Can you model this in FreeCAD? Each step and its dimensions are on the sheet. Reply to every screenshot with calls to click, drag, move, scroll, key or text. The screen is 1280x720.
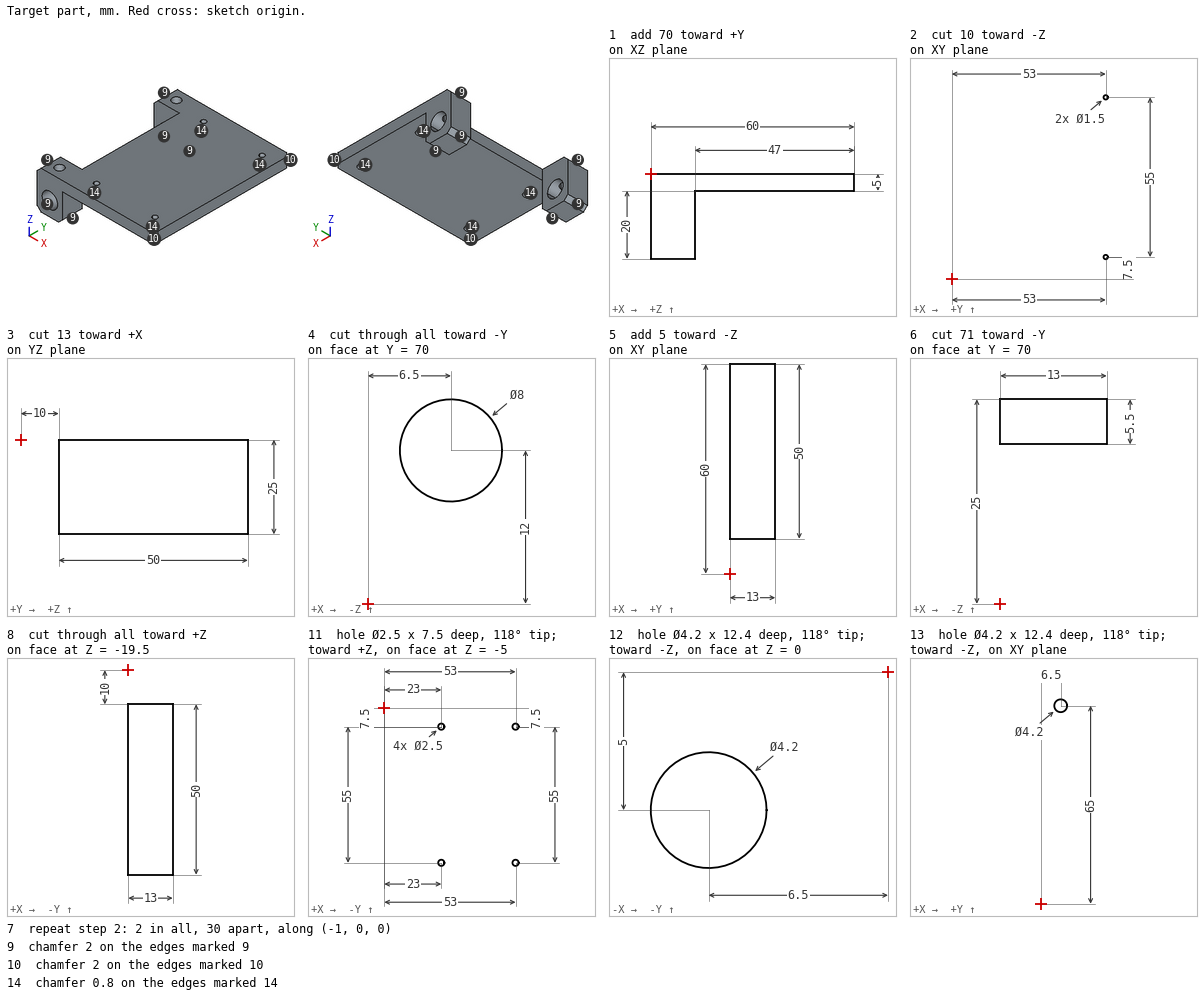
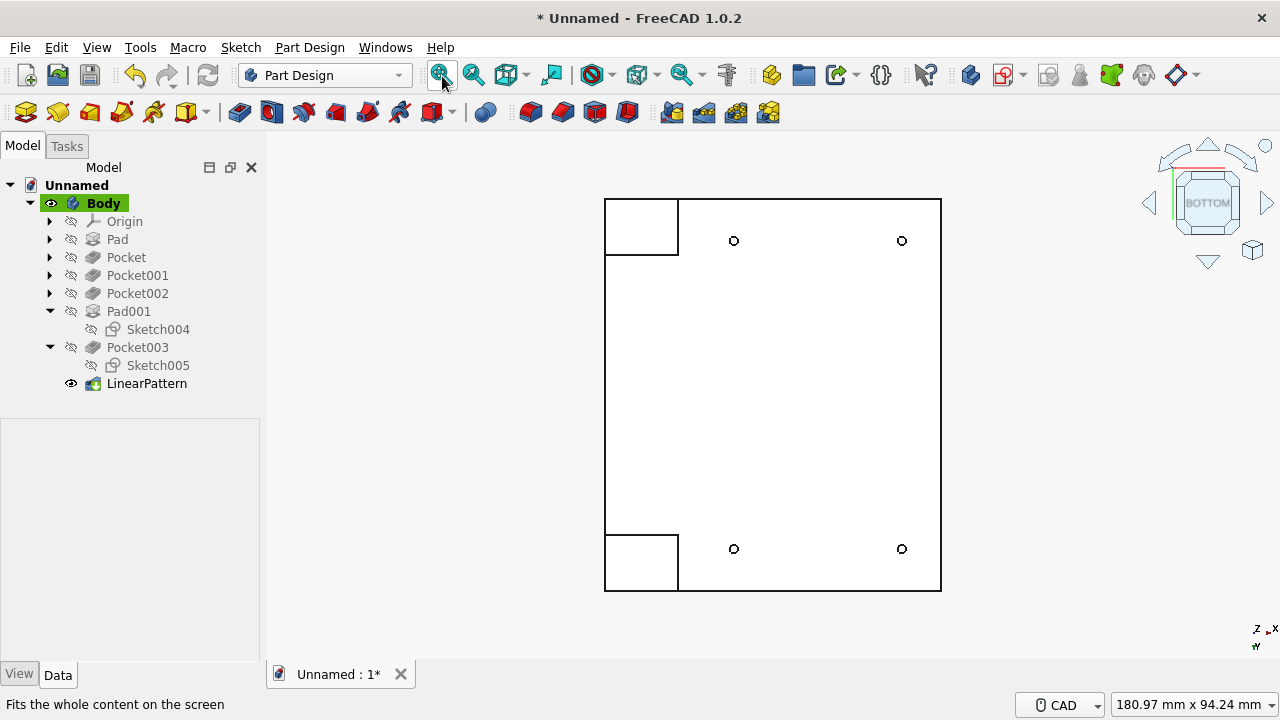
click(641, 562)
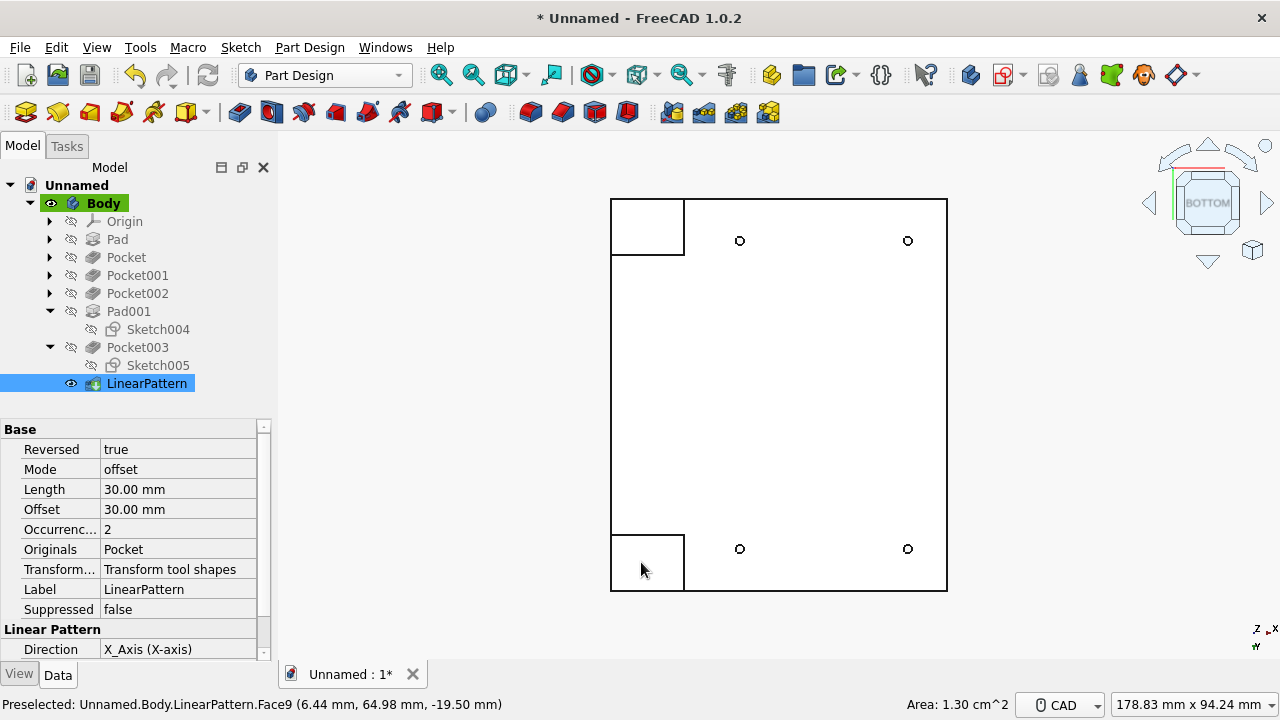
click(1004, 76)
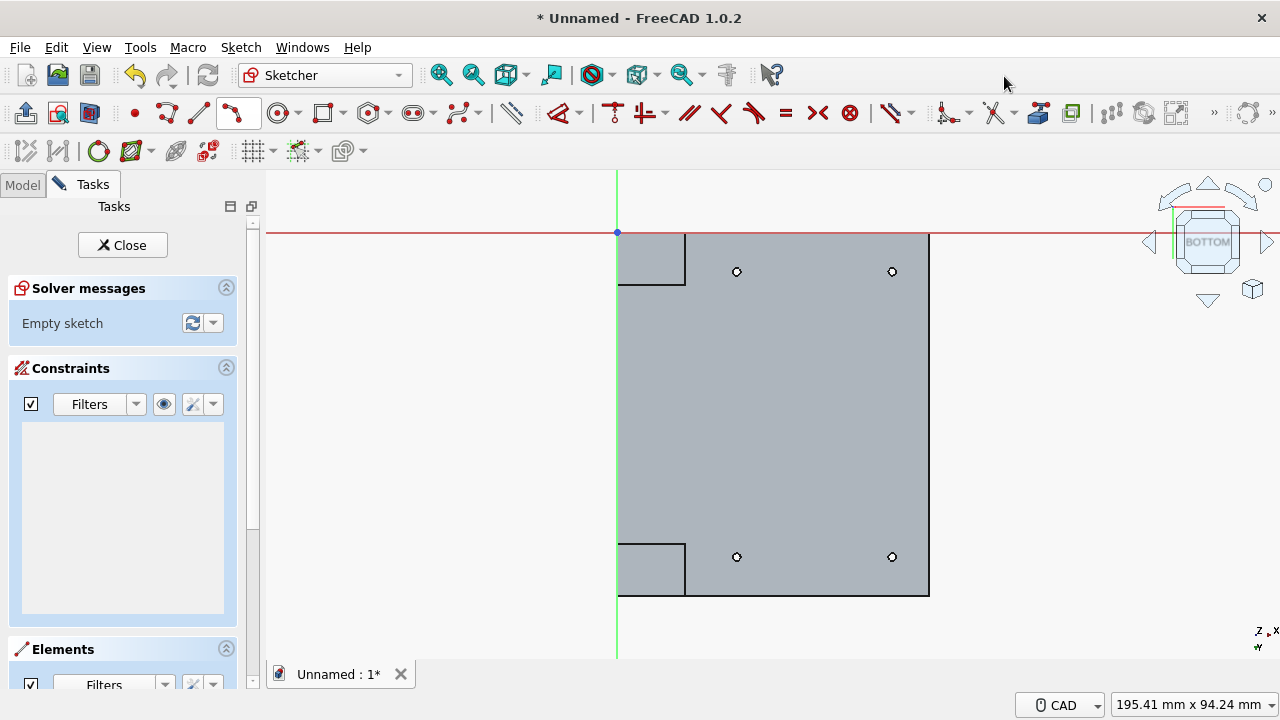
key(g)
key(r)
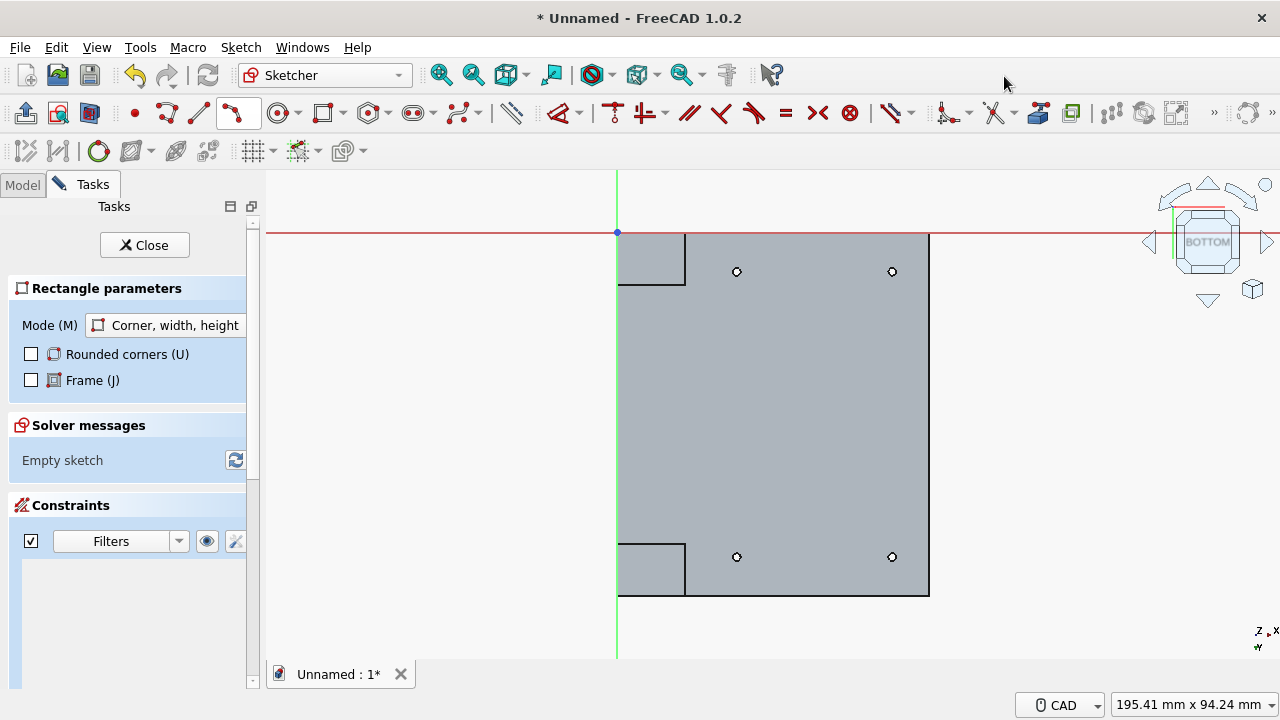
click(617, 285)
move(685, 544)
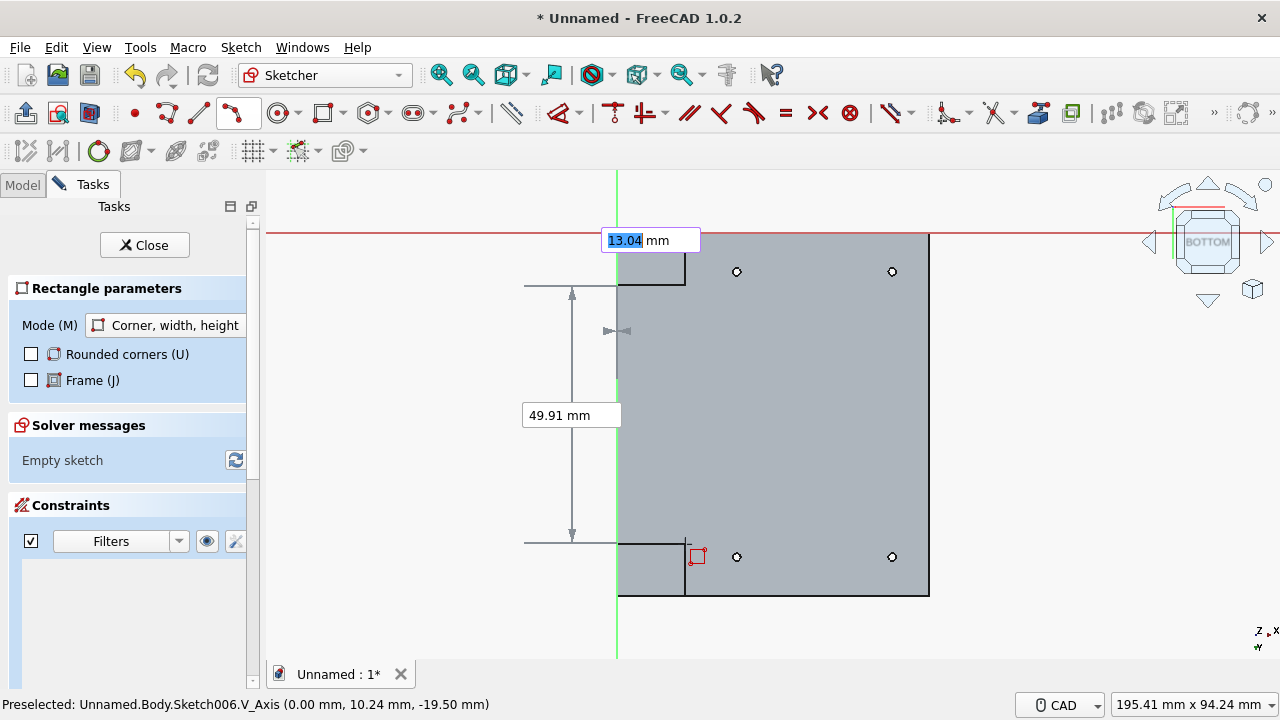
text(13)
key(Tab)
text(50)
key(Return)
key(Escape)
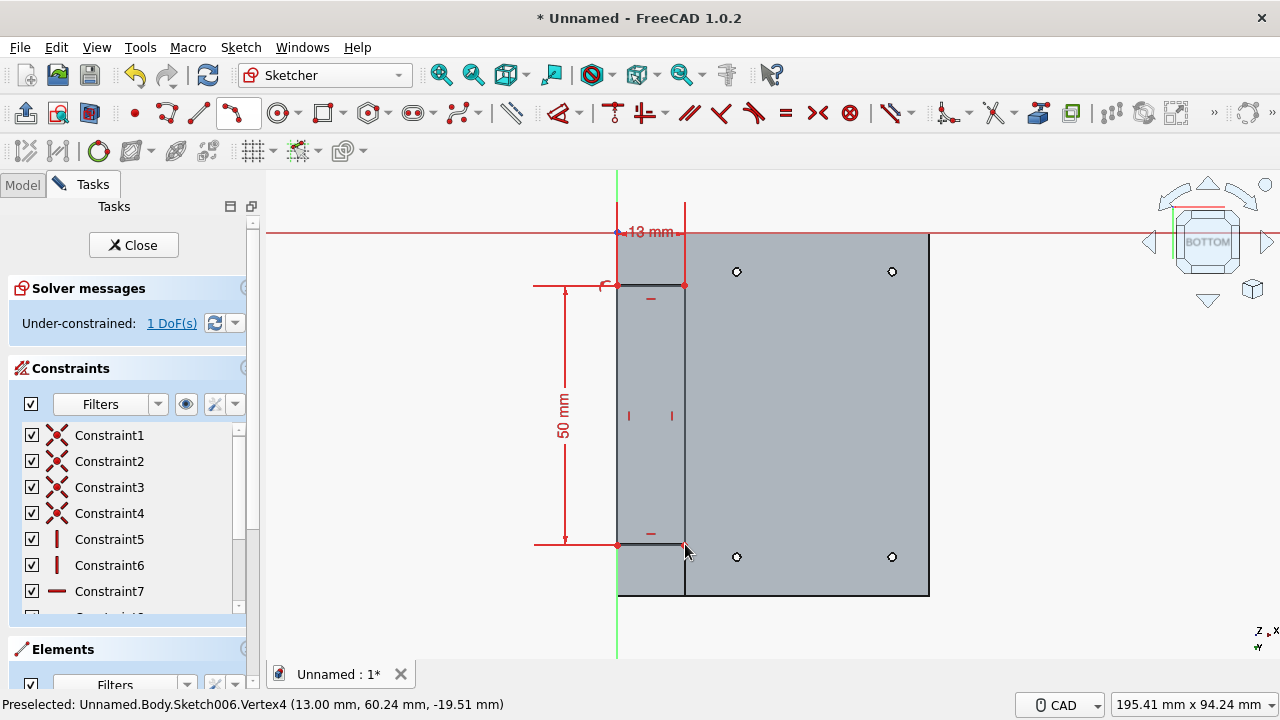
key(d)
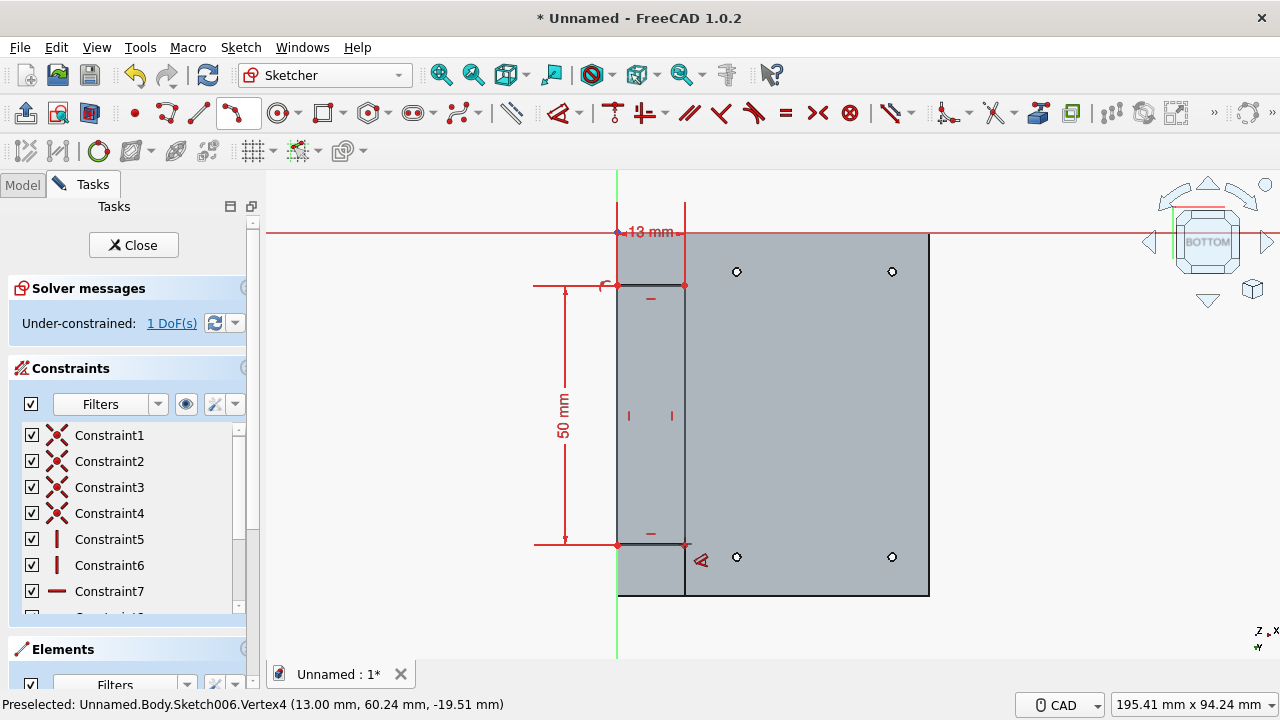
click(617, 286)
click(583, 259)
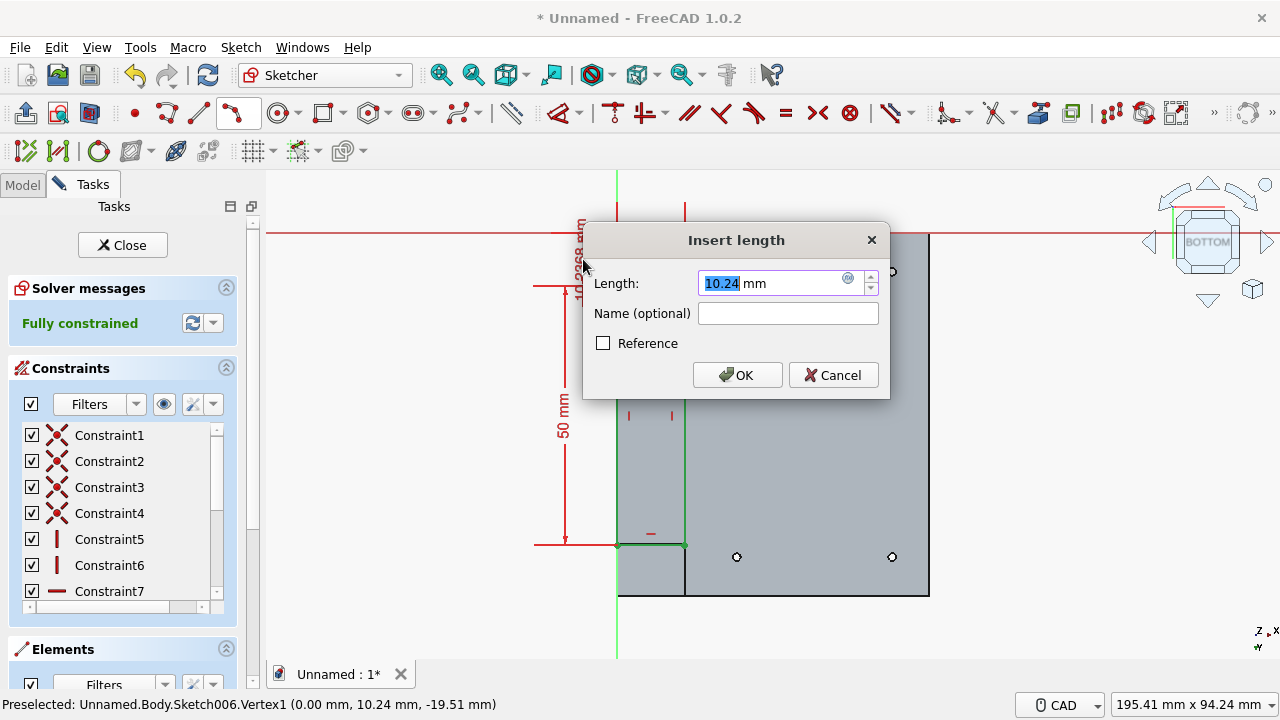
text(10)
key(Return)
key(Escape)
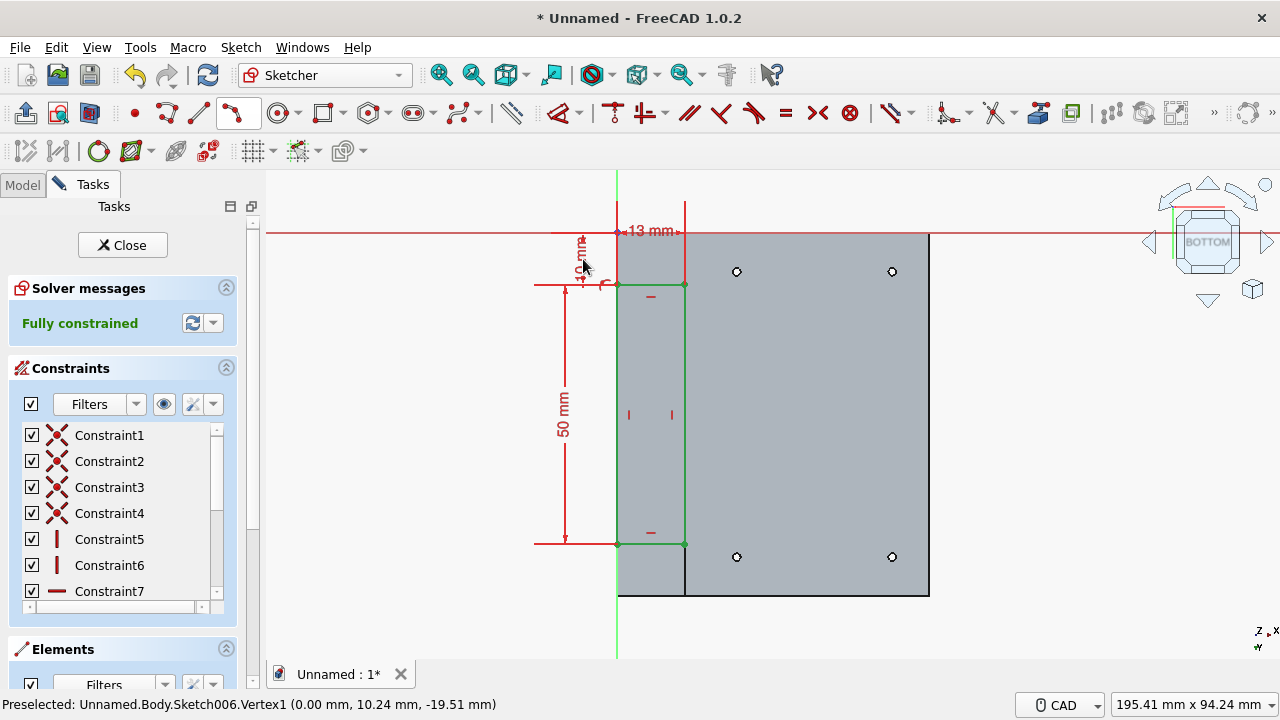
click(123, 245)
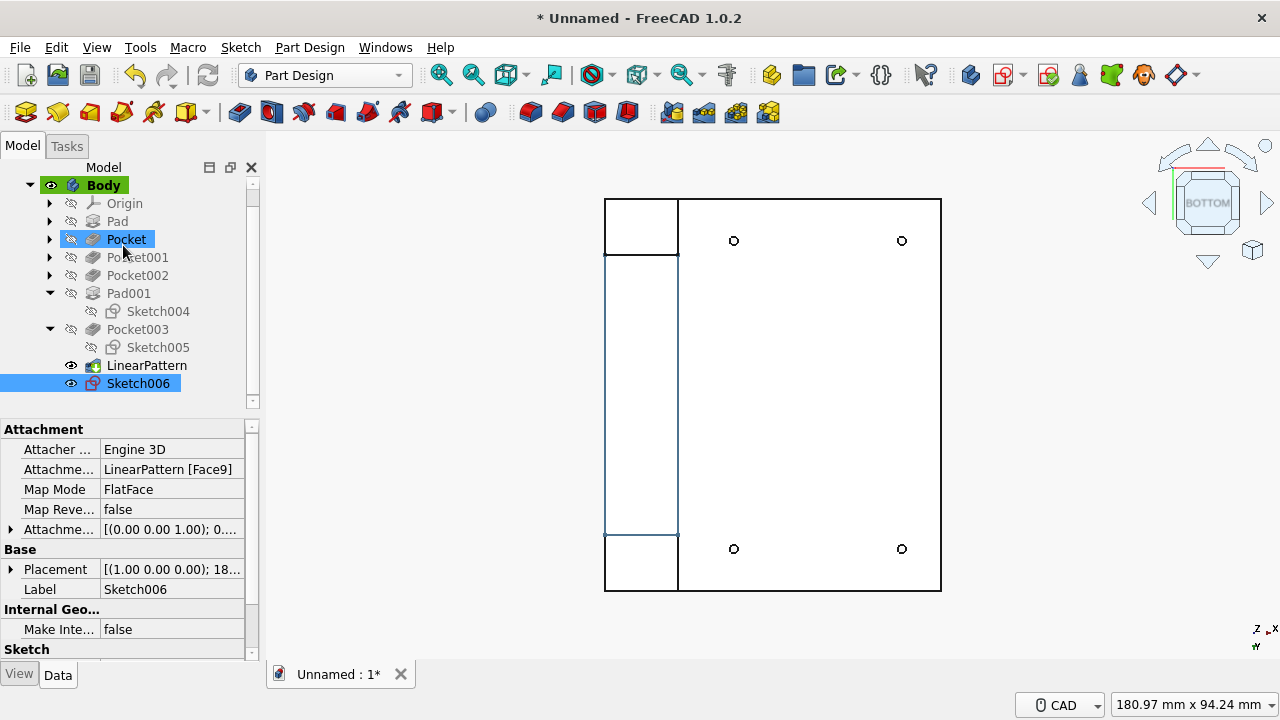
click(240, 112)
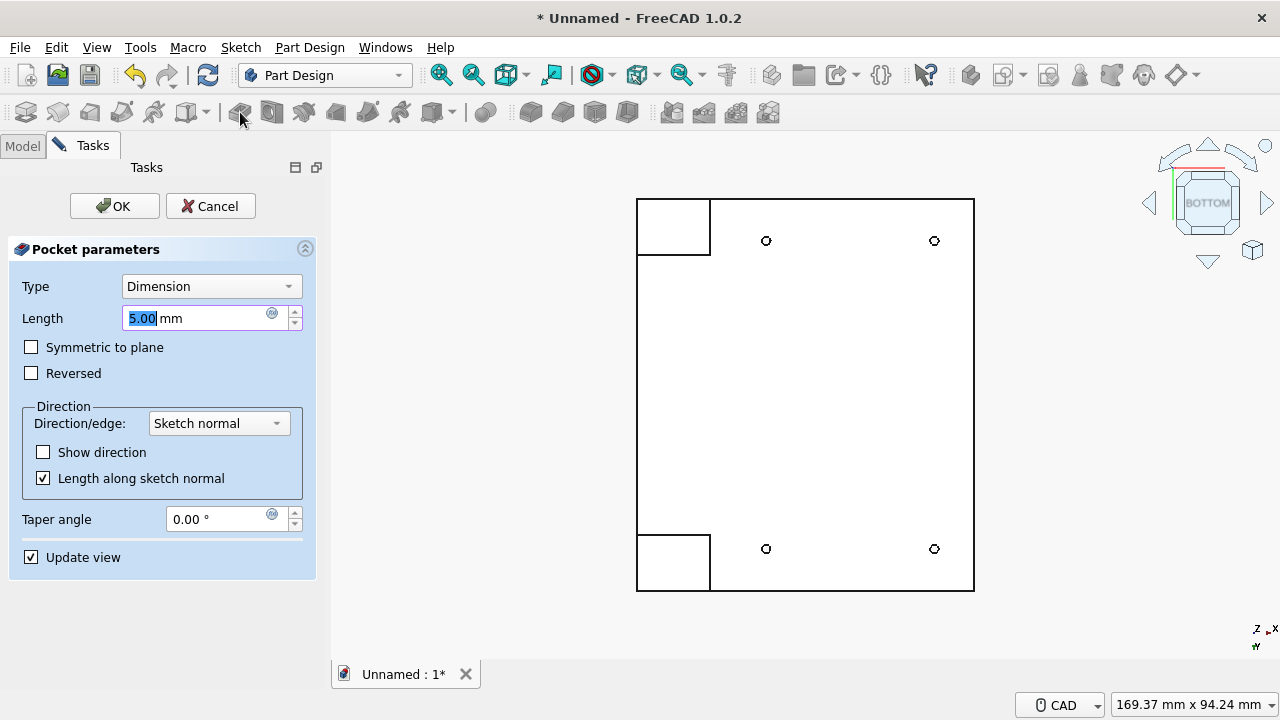
click(212, 286)